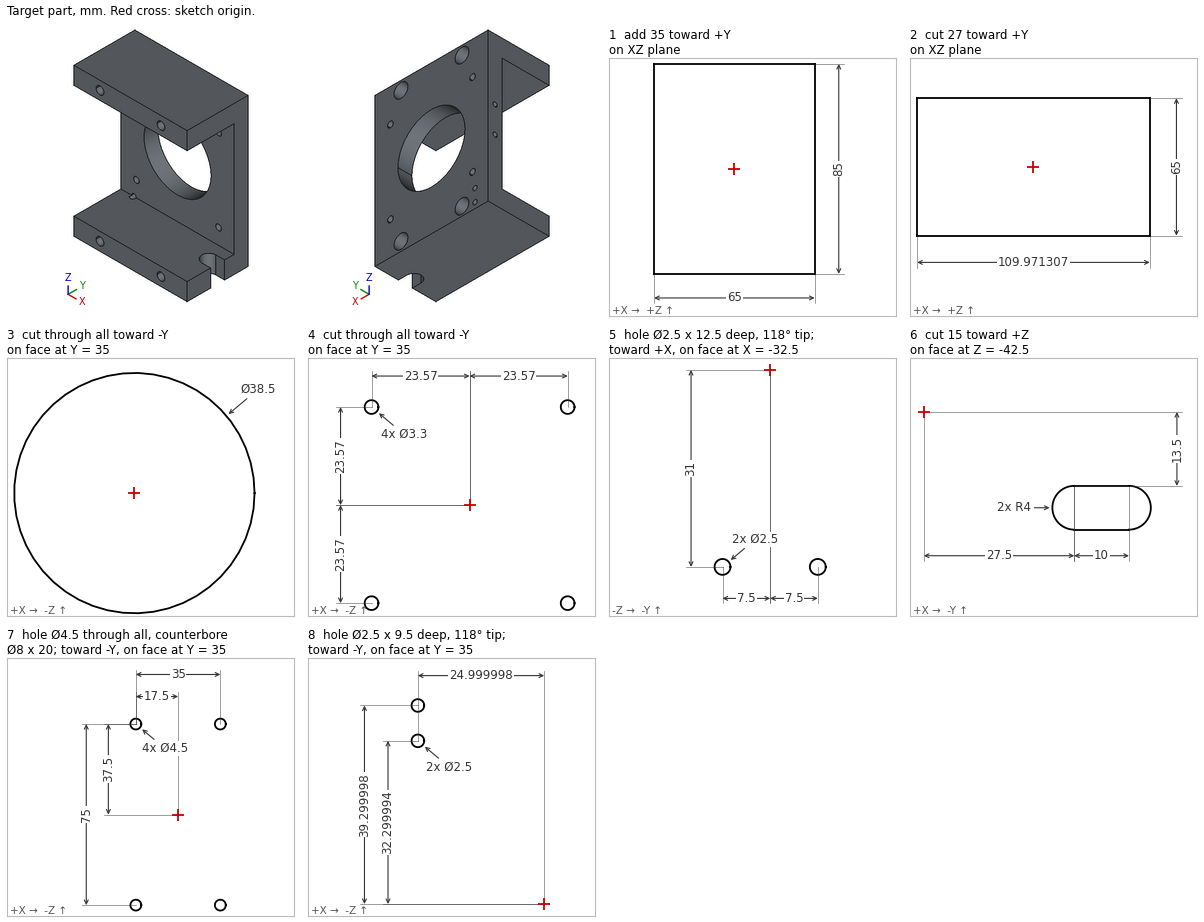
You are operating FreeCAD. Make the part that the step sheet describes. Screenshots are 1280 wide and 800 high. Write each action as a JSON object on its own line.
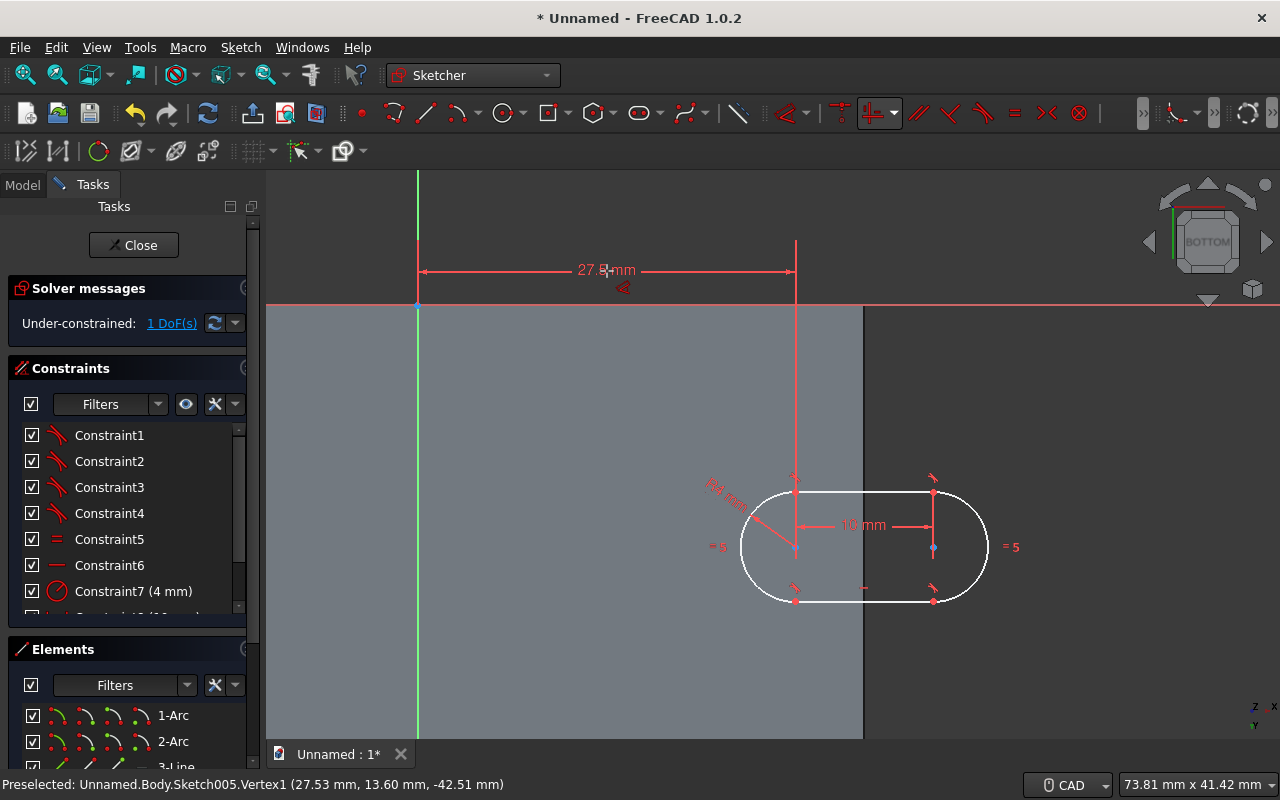
{"action": "left_click", "coordinate": [796, 492]}
{"action": "left_click", "coordinate": [384, 399]}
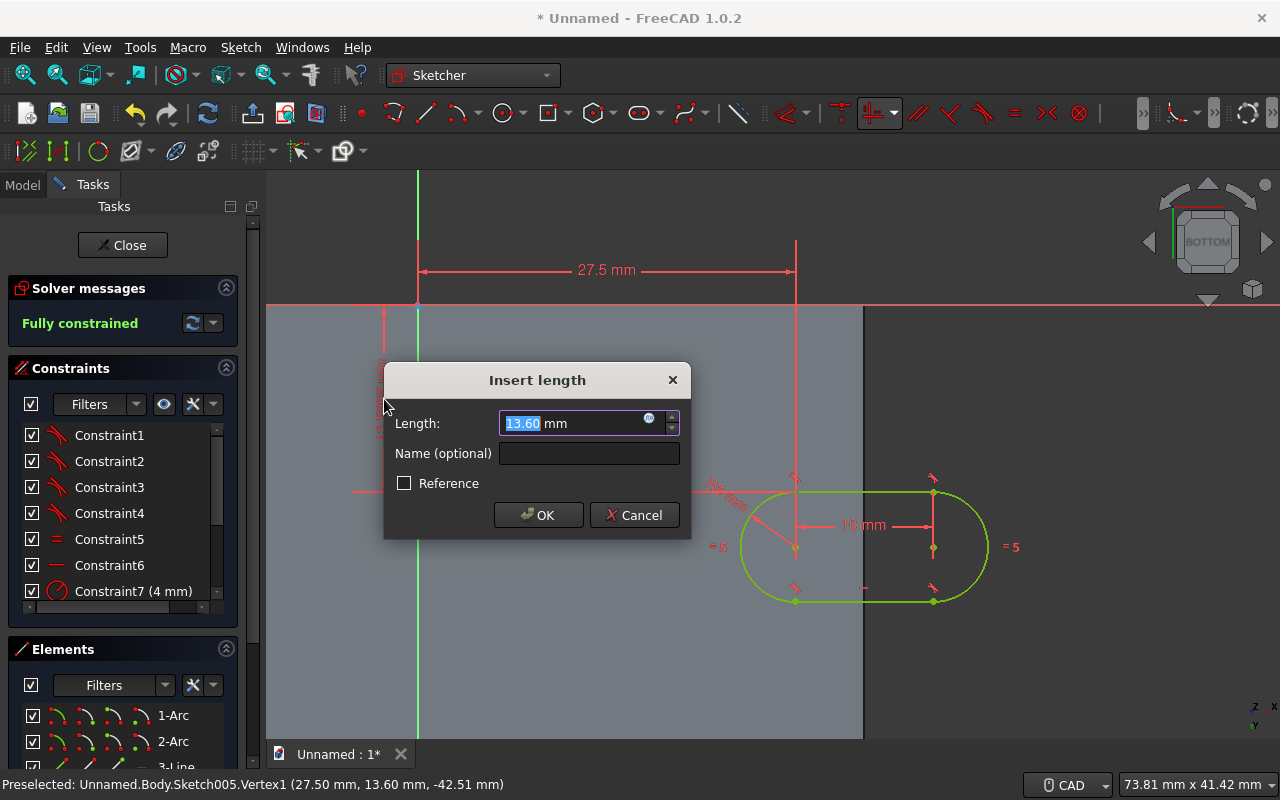
{"action": "type", "text": "13.5"}
{"action": "key", "text": "Return"}
{"action": "key", "text": "Escape"}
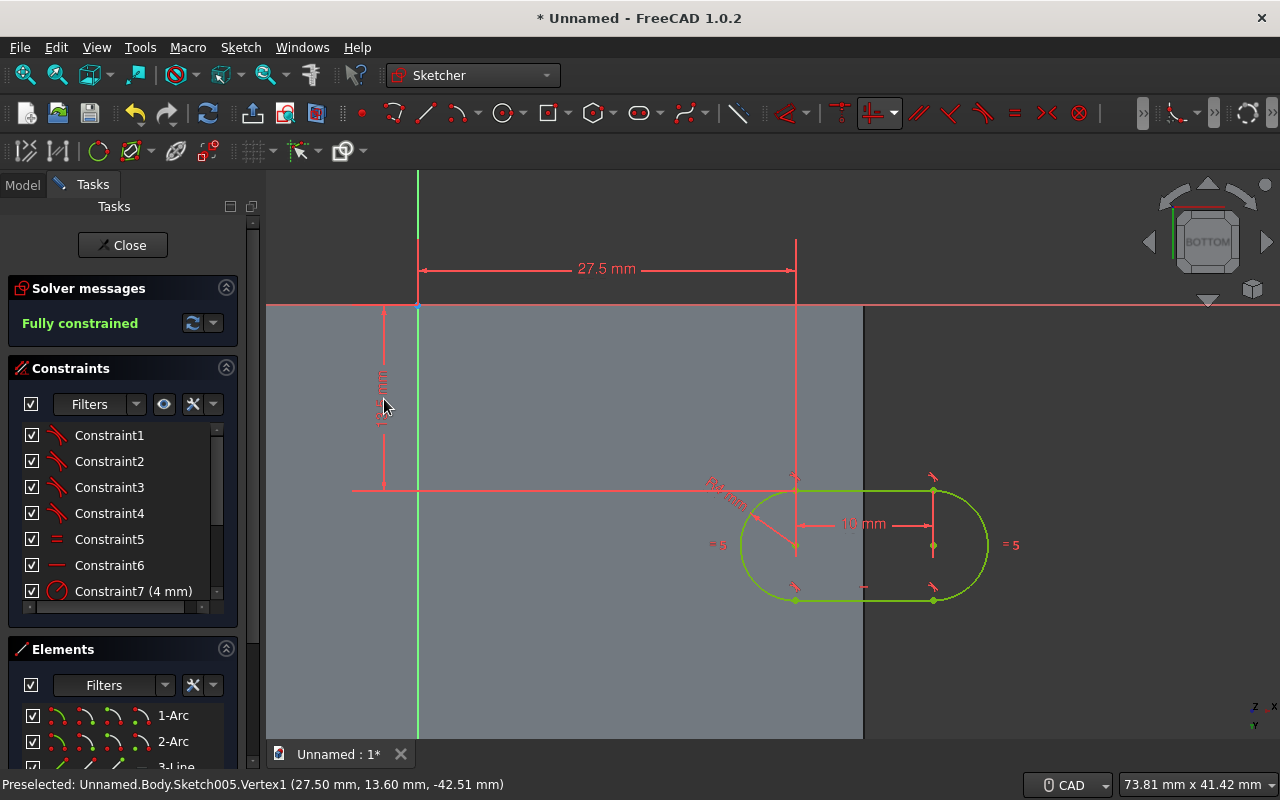
{"action": "left_click", "coordinate": [123, 245]}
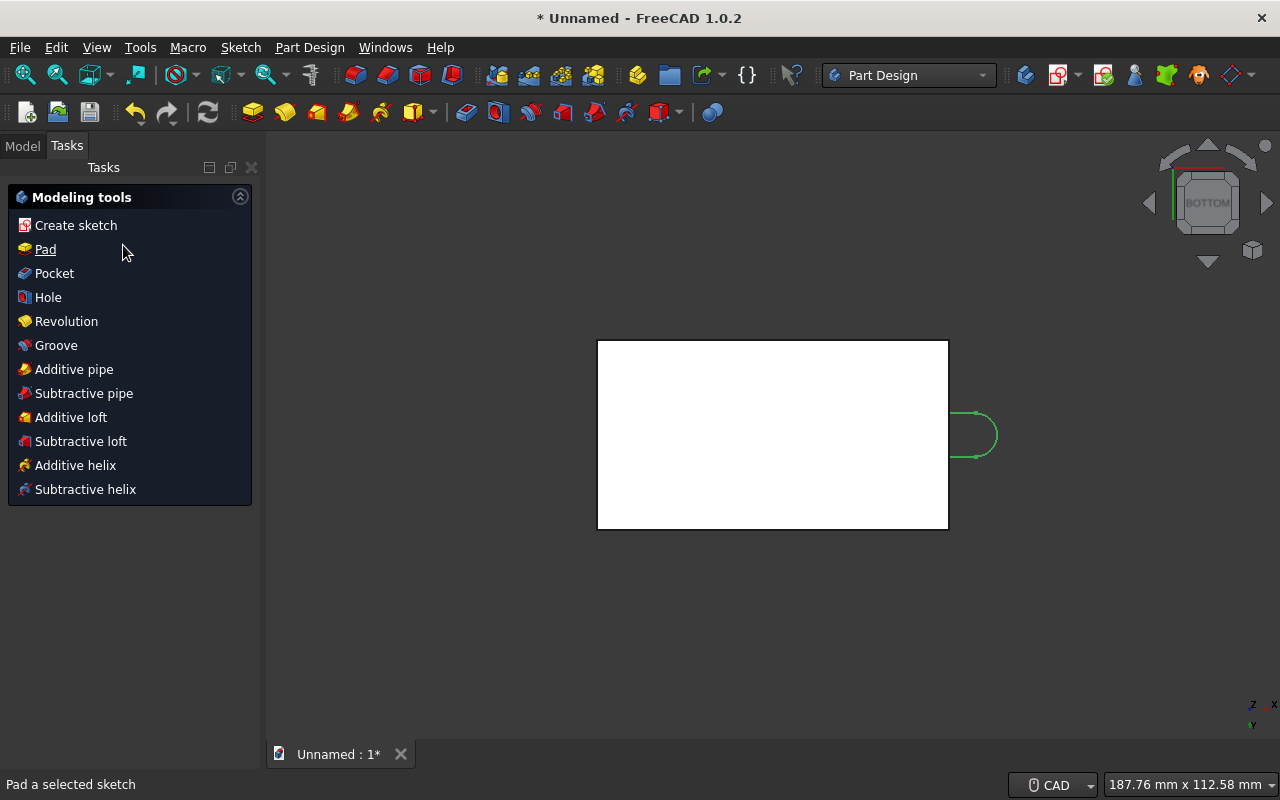
{"action": "left_click", "coordinate": [468, 112]}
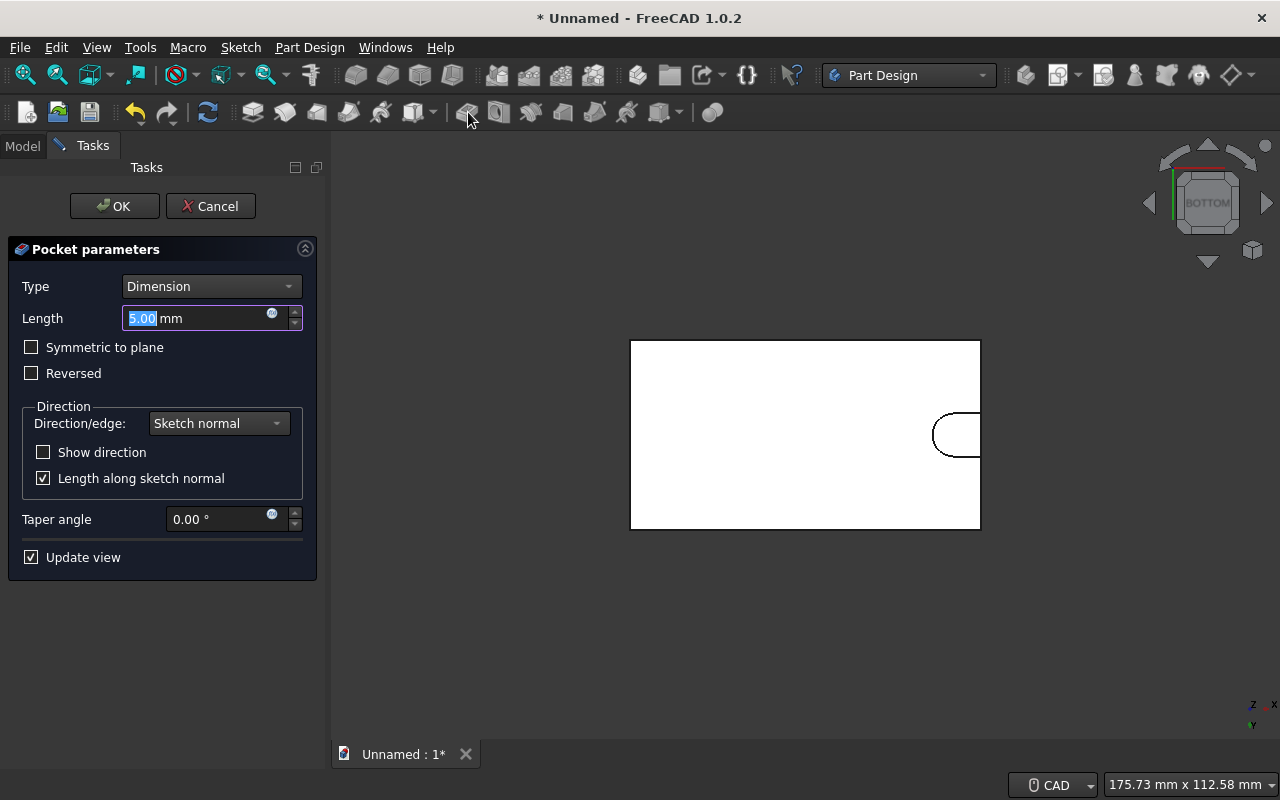
{"action": "type", "text": "15"}
{"action": "key", "text": "Tab"}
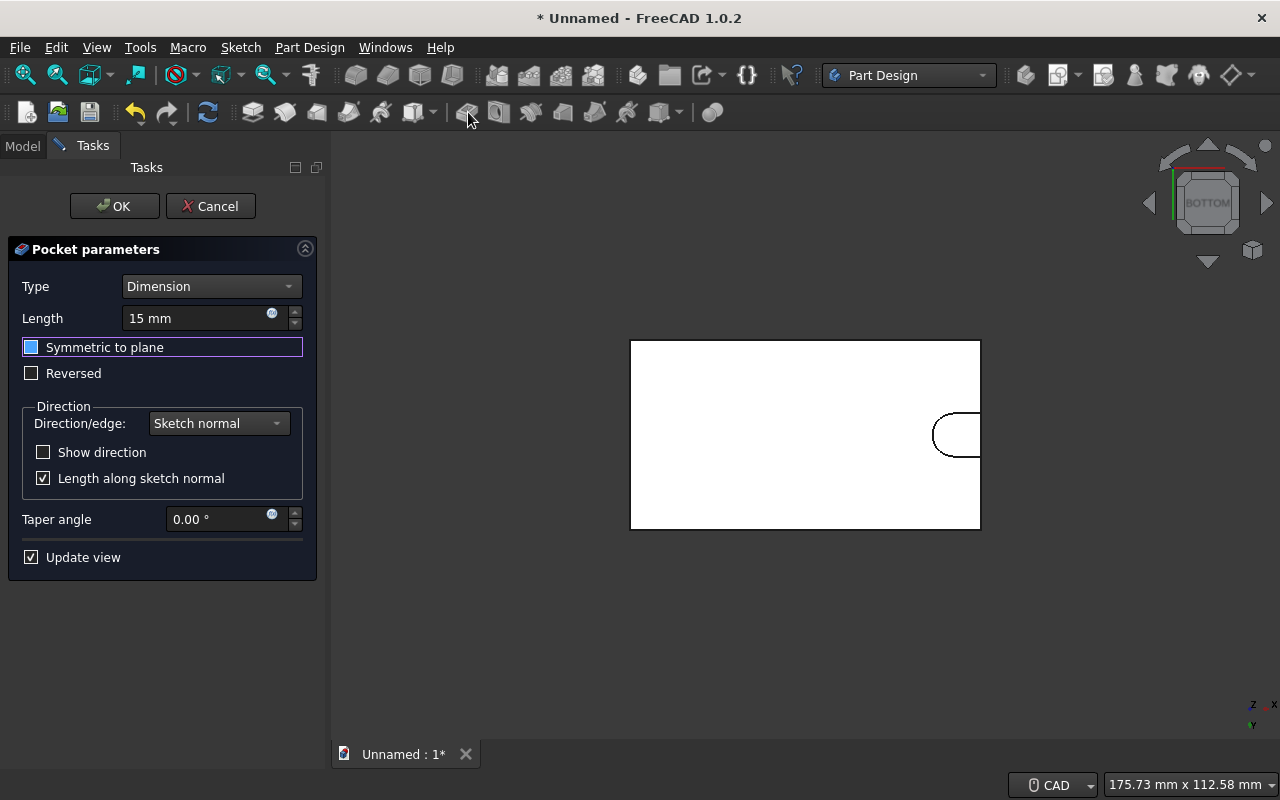
{"action": "left_click", "coordinate": [115, 206]}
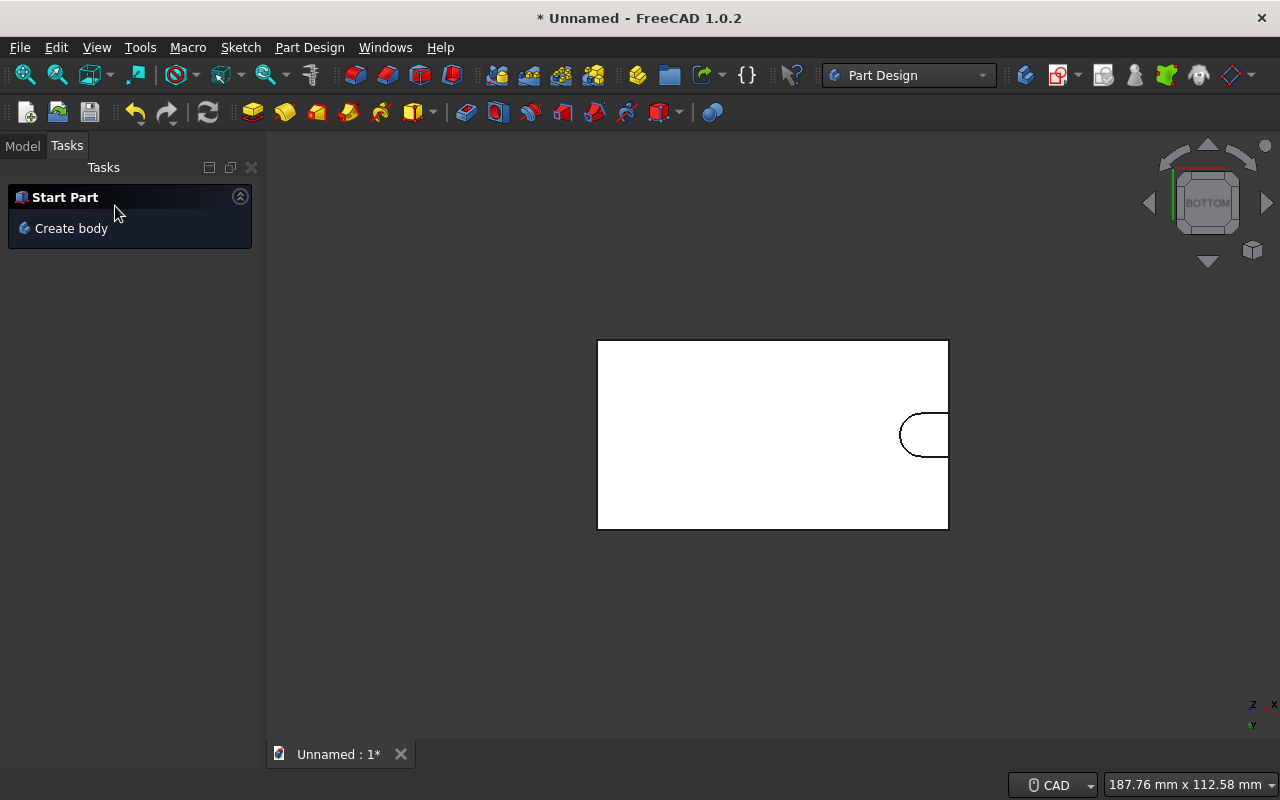
{"action": "left_click", "coordinate": [26, 76]}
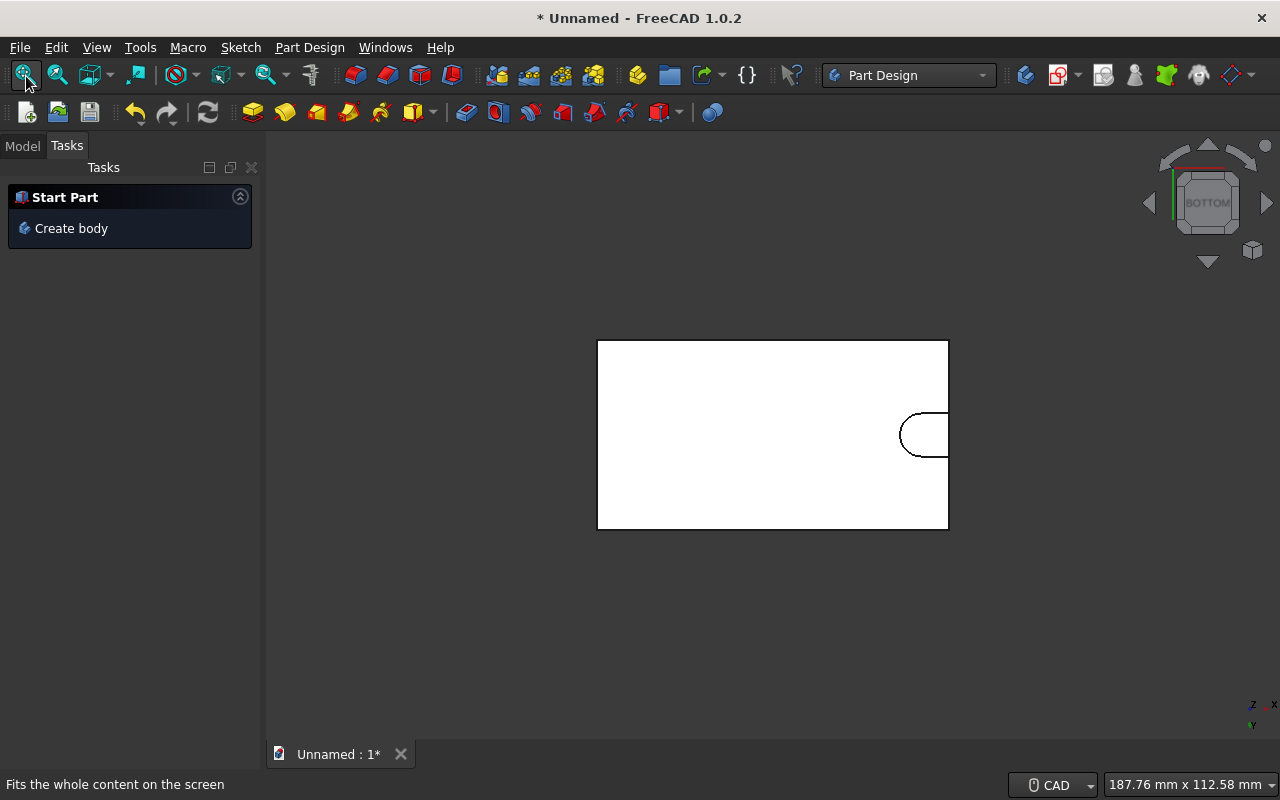
{"action": "key", "text": "4"}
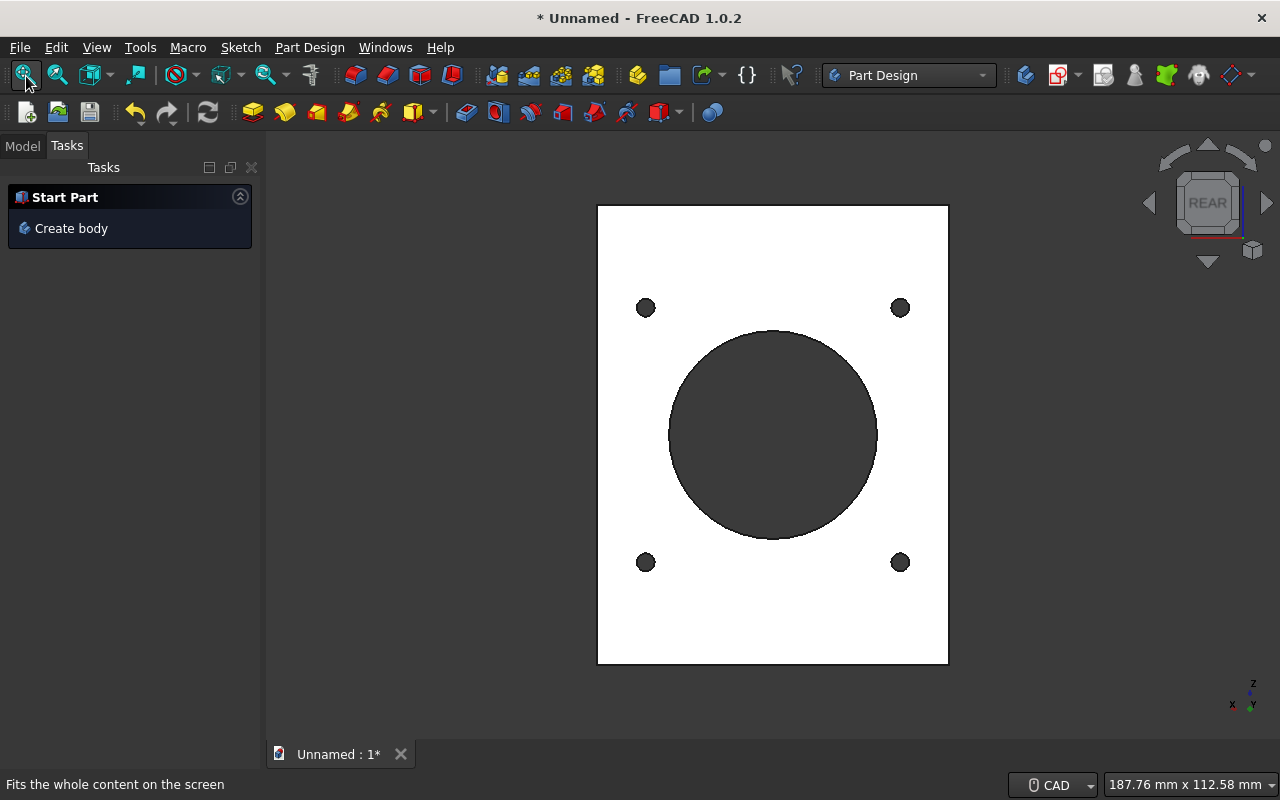
{"action": "left_click", "coordinate": [723, 565]}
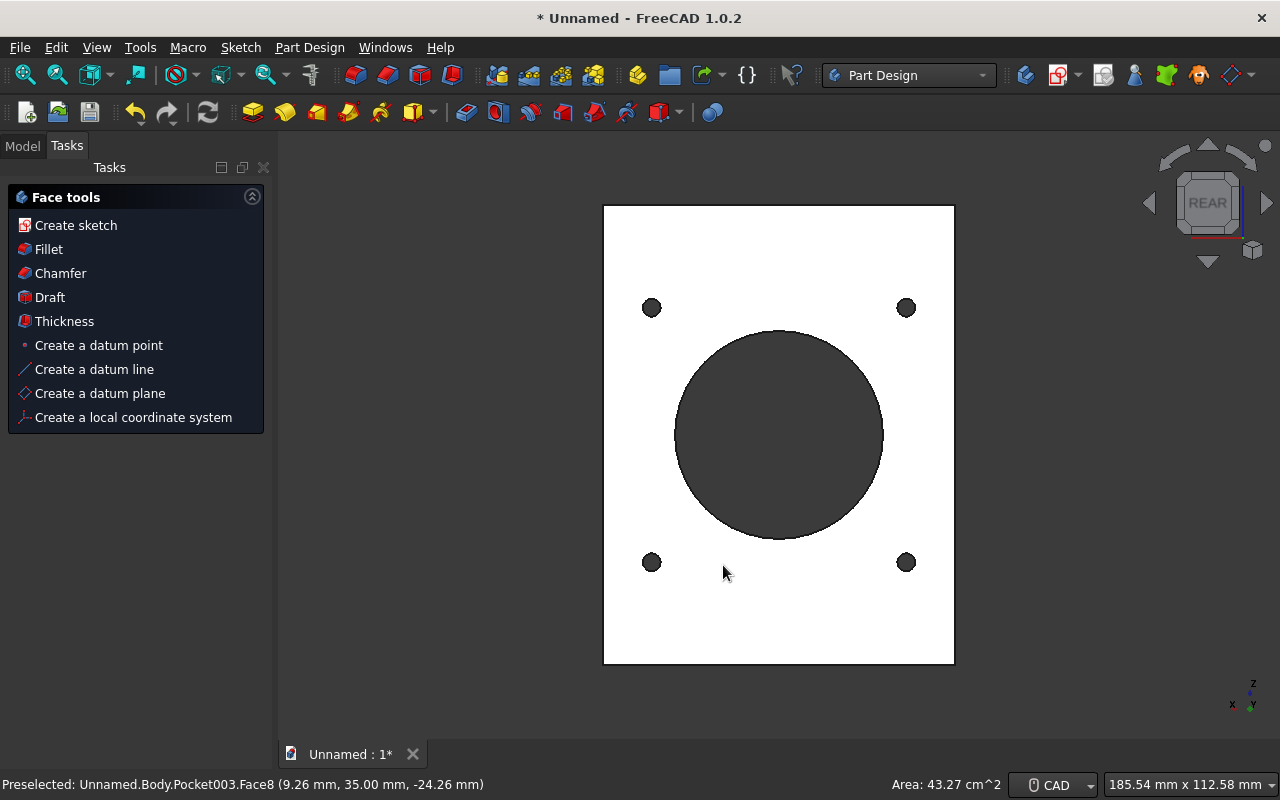
{"action": "left_click", "coordinate": [1058, 76]}